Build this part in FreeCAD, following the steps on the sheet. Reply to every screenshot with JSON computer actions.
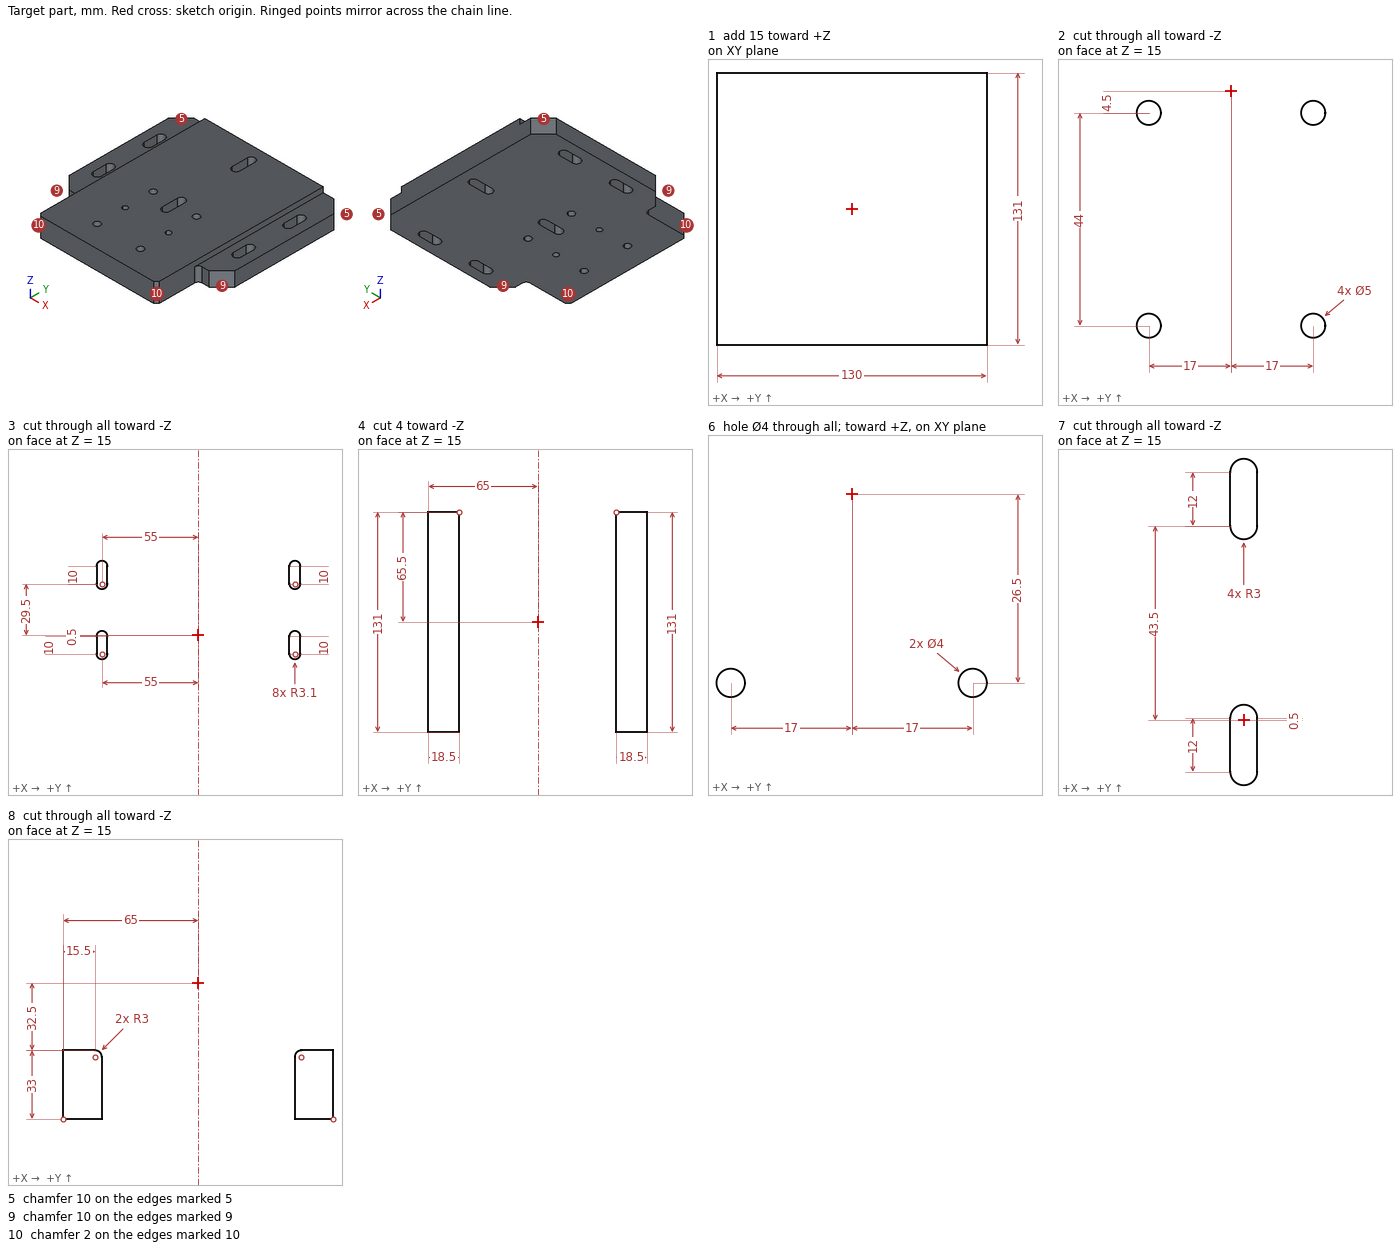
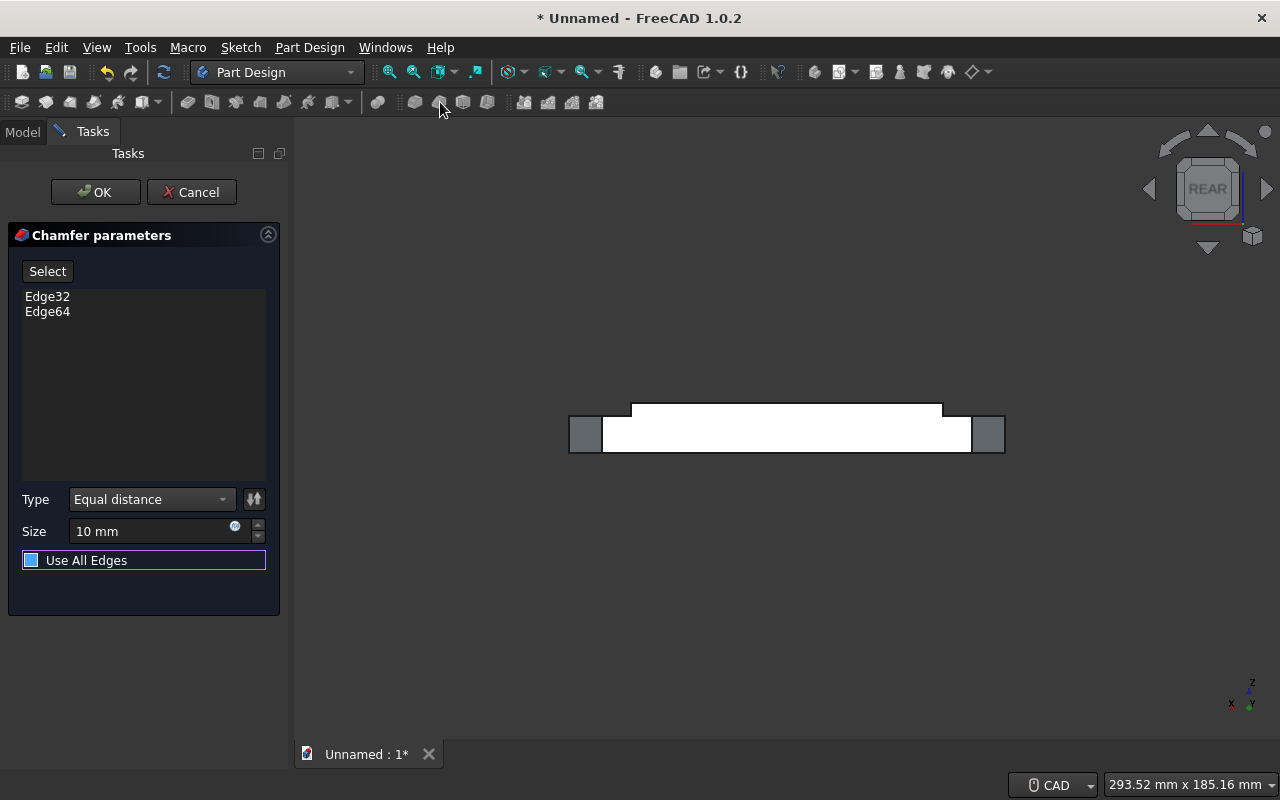
{"action": "left_click", "coordinate": [96, 192]}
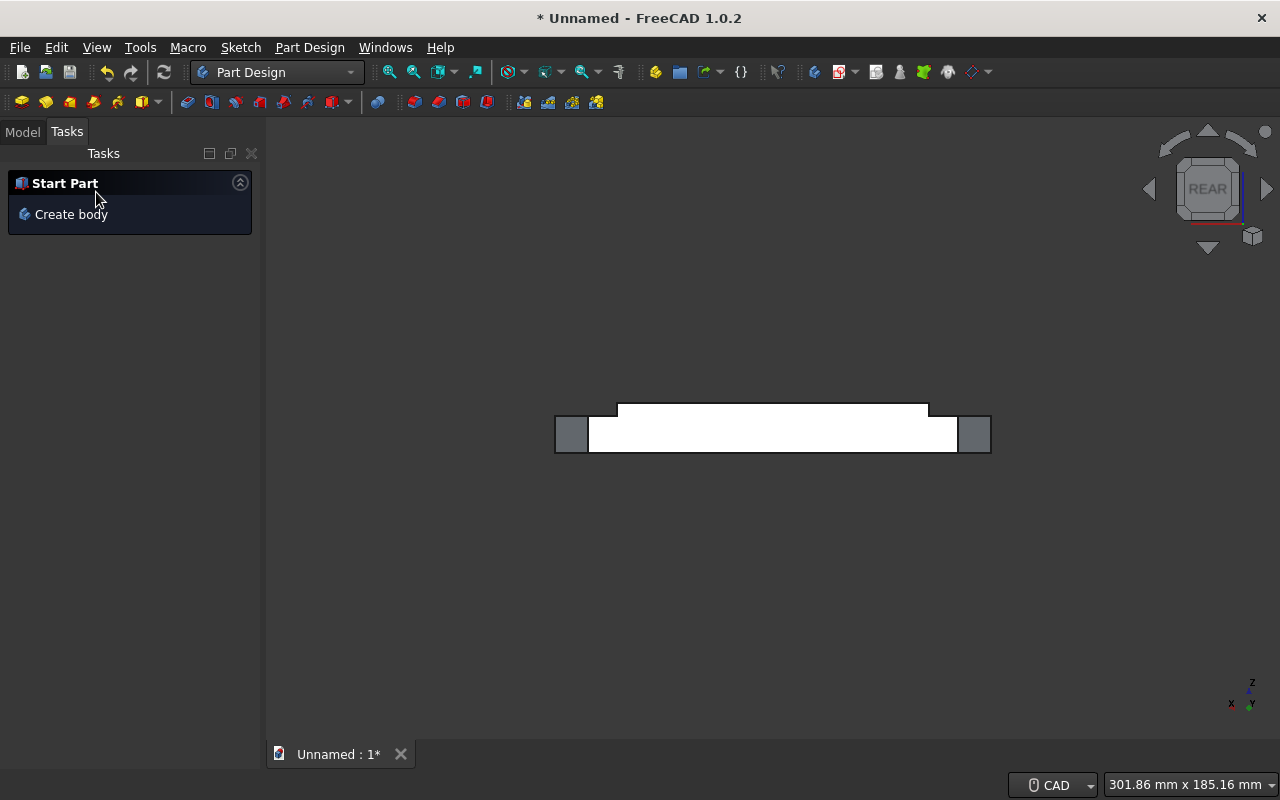
{"action": "key", "text": "v f"}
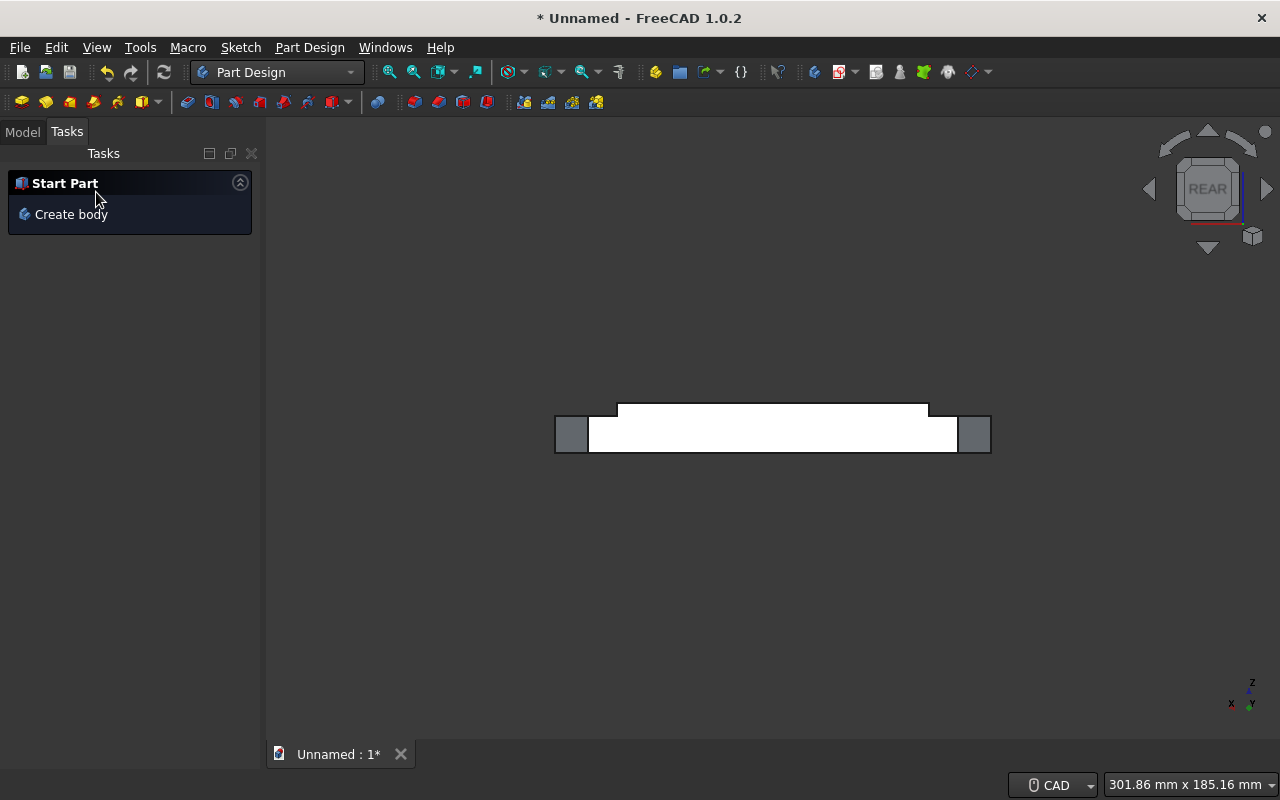
{"action": "left_click", "coordinate": [840, 72]}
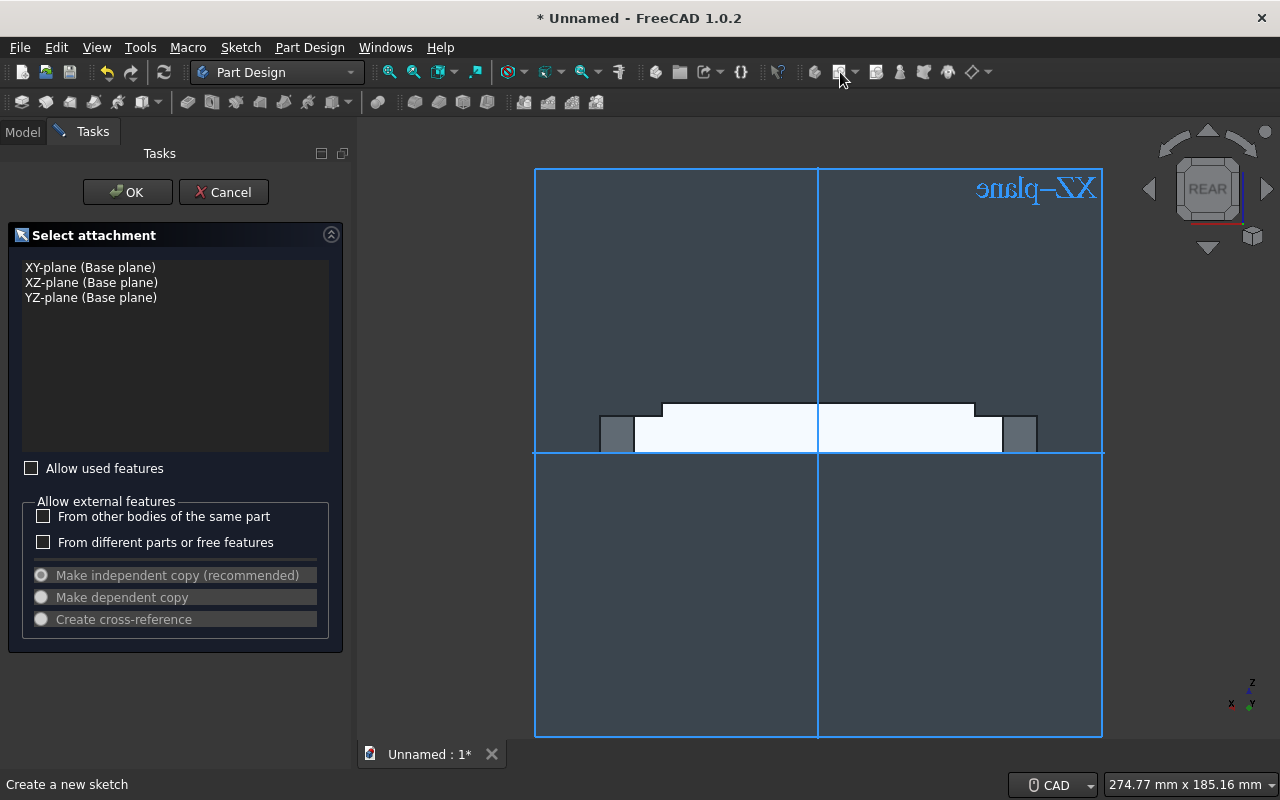
{"action": "left_click", "coordinate": [82, 268]}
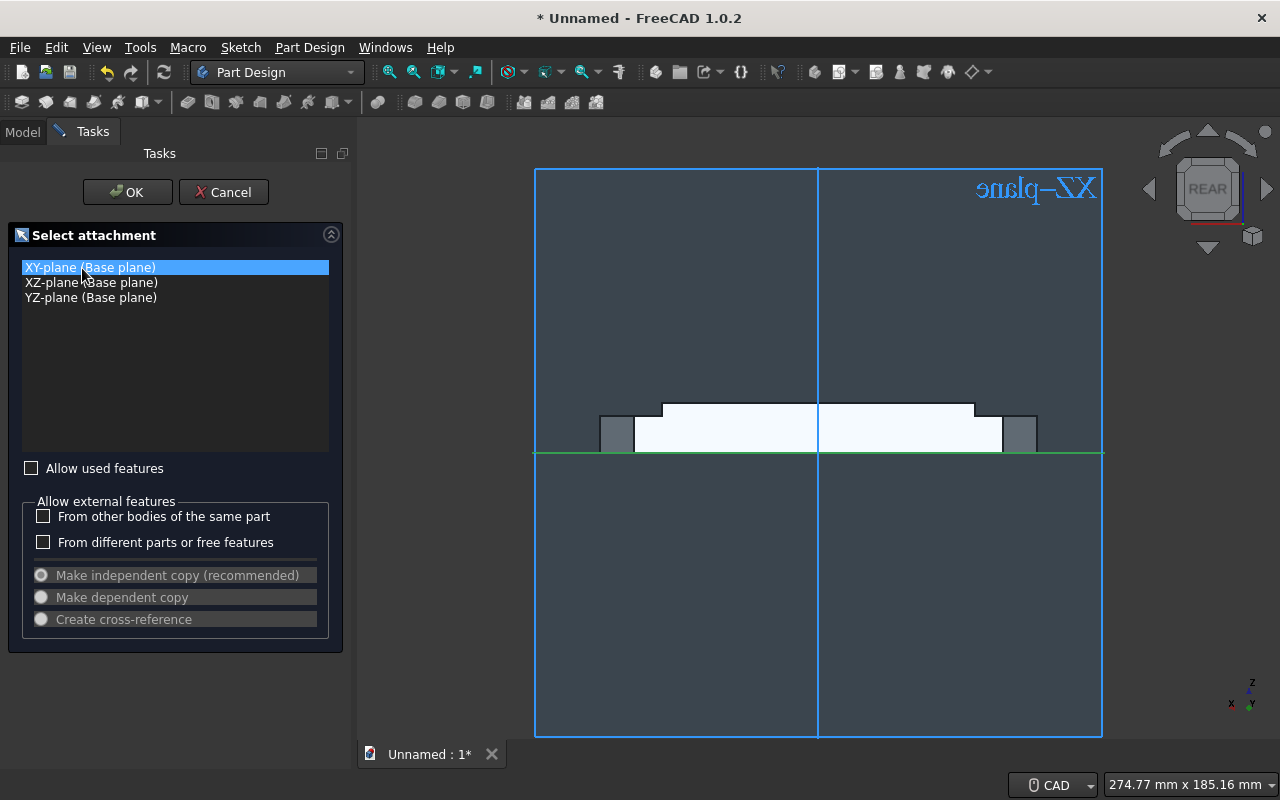
{"action": "left_click", "coordinate": [128, 192]}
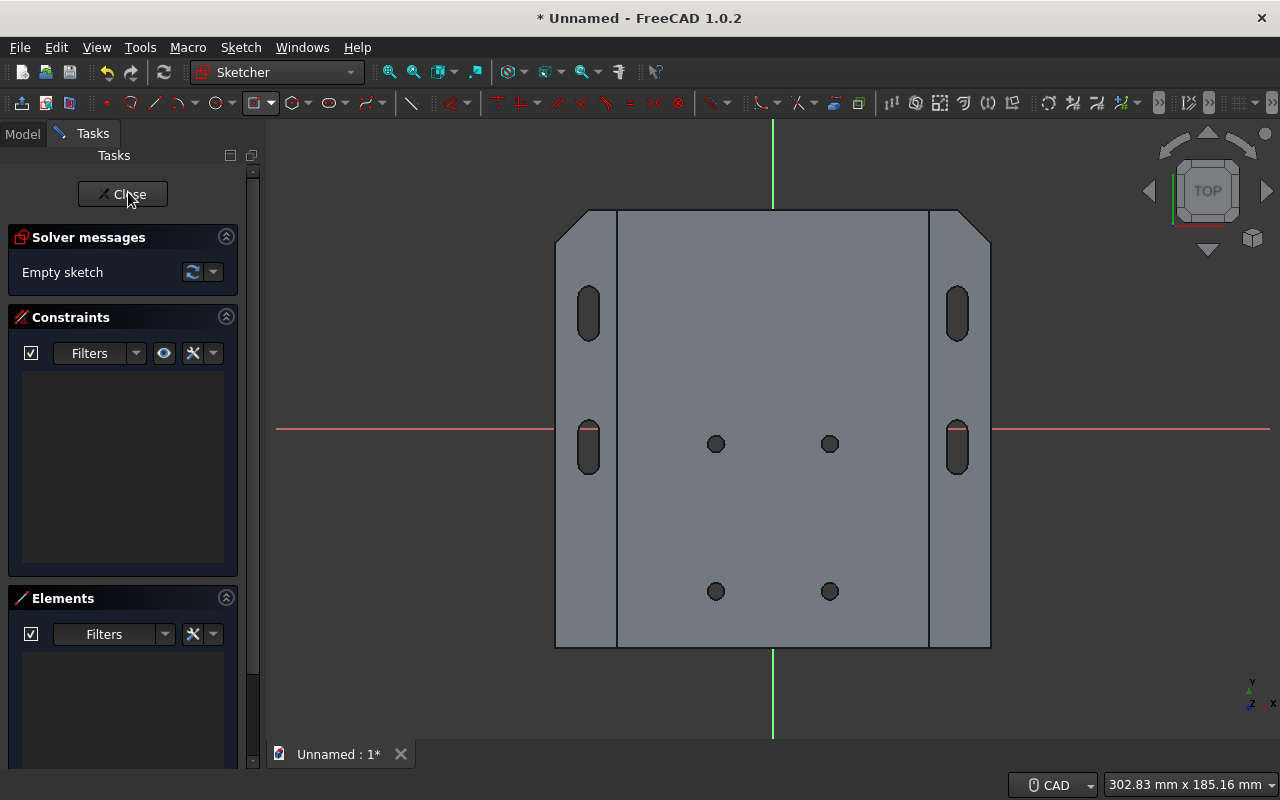
{"action": "key", "text": "q s"}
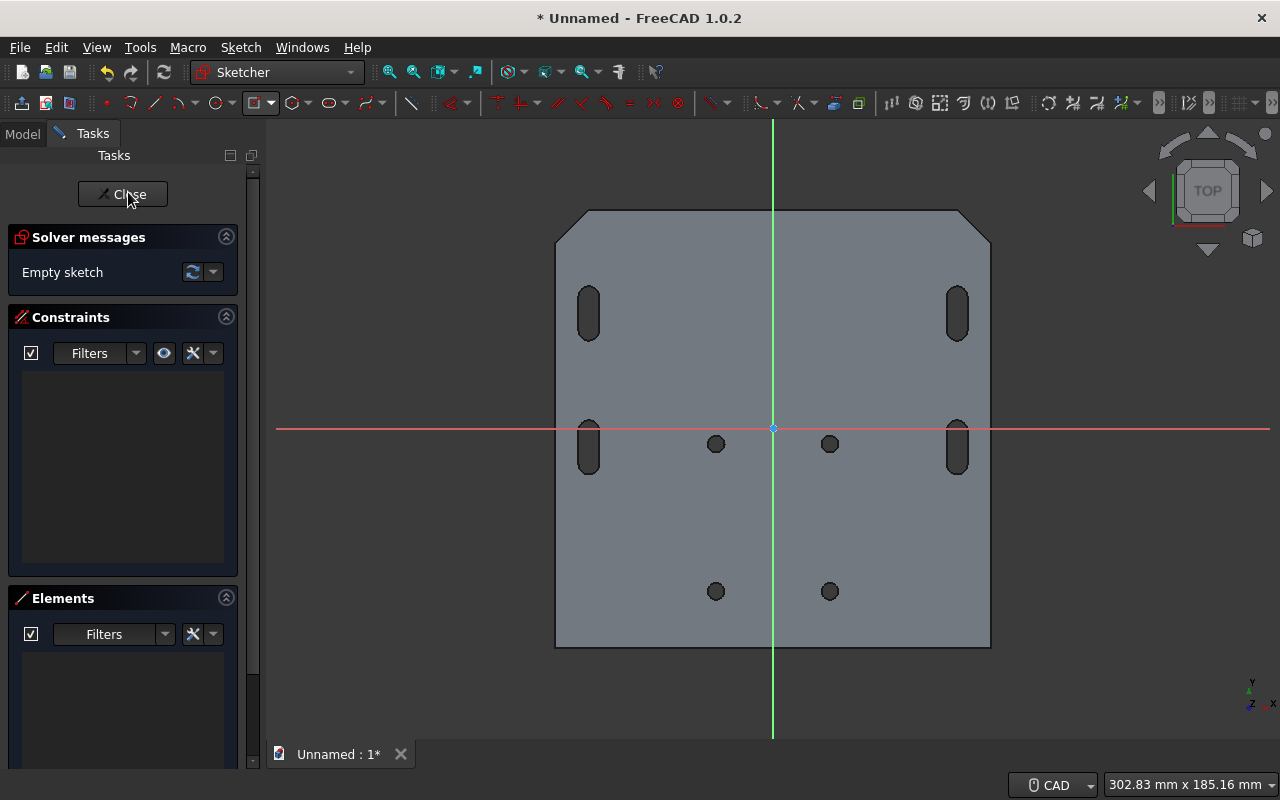
{"action": "scroll", "coordinate": [795, 492], "scroll_direction": "up", "scroll_amount": 7}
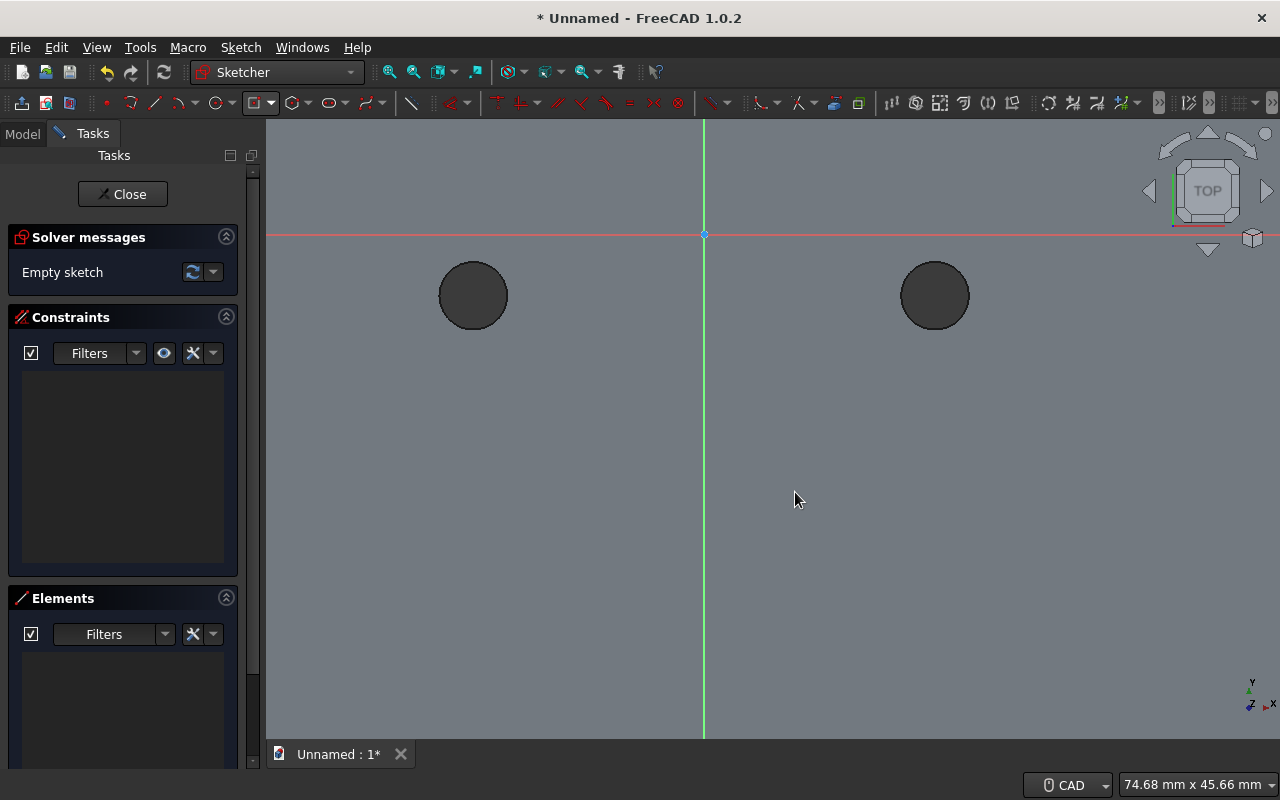
{"action": "key", "text": "g c"}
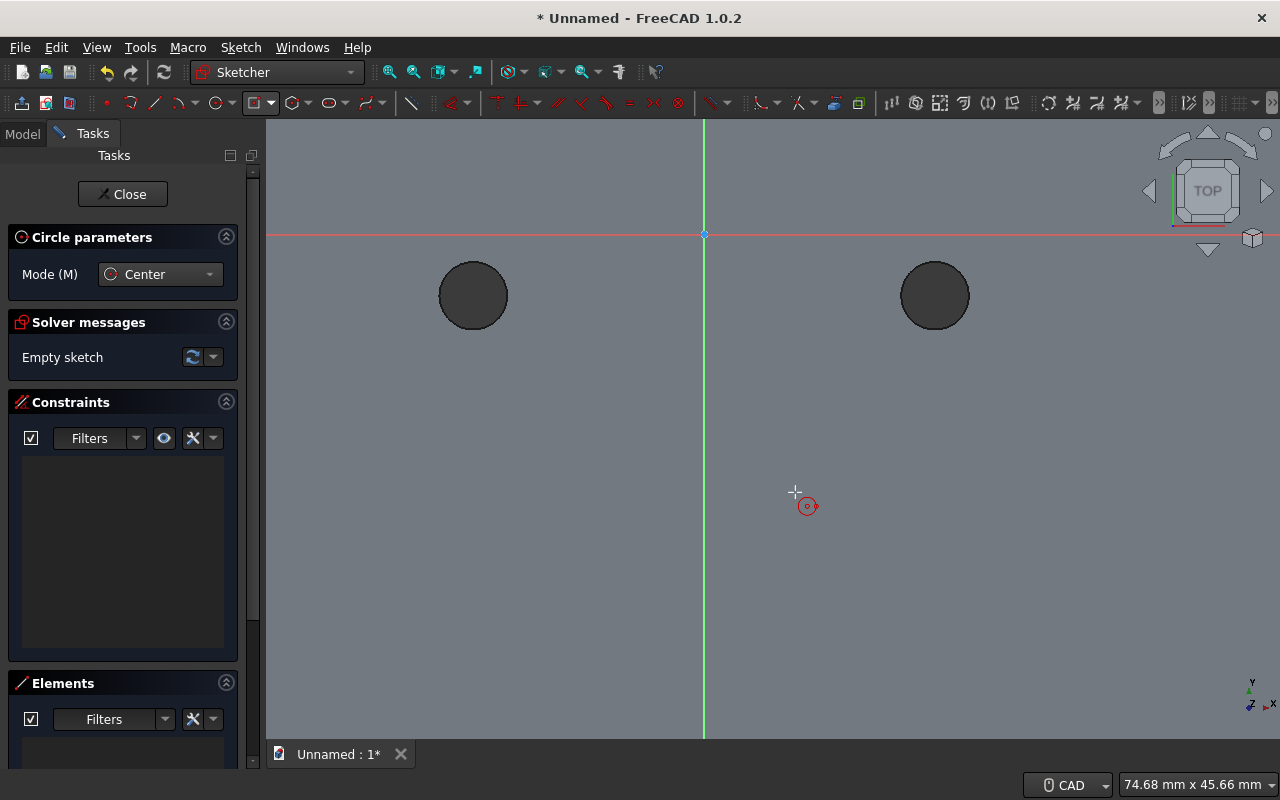
{"action": "left_click", "coordinate": [935, 595]}
{"action": "mouse_move", "coordinate": [954, 575]}